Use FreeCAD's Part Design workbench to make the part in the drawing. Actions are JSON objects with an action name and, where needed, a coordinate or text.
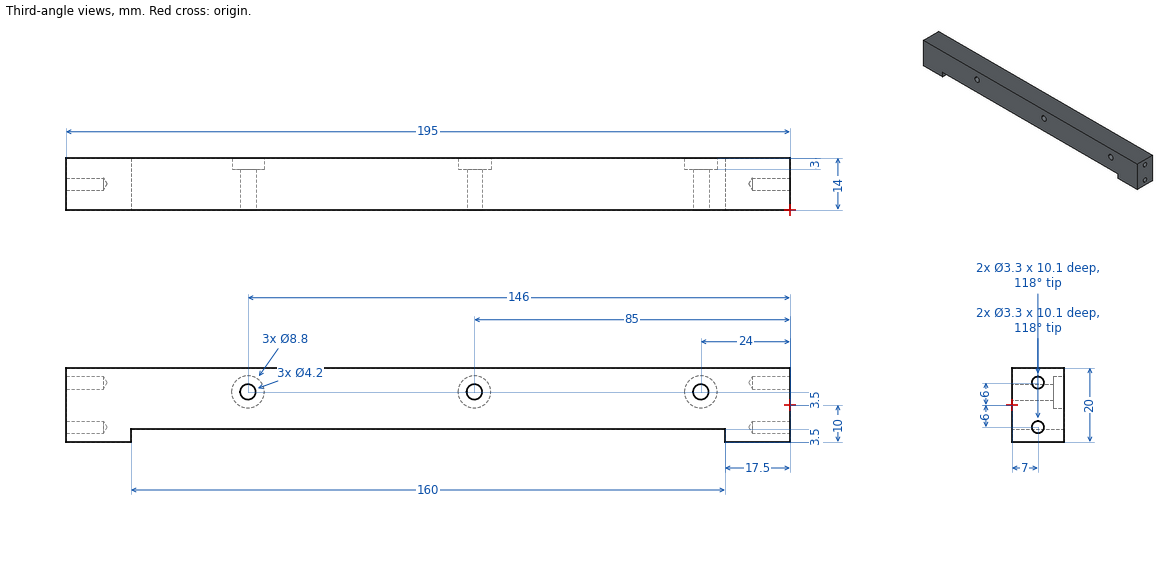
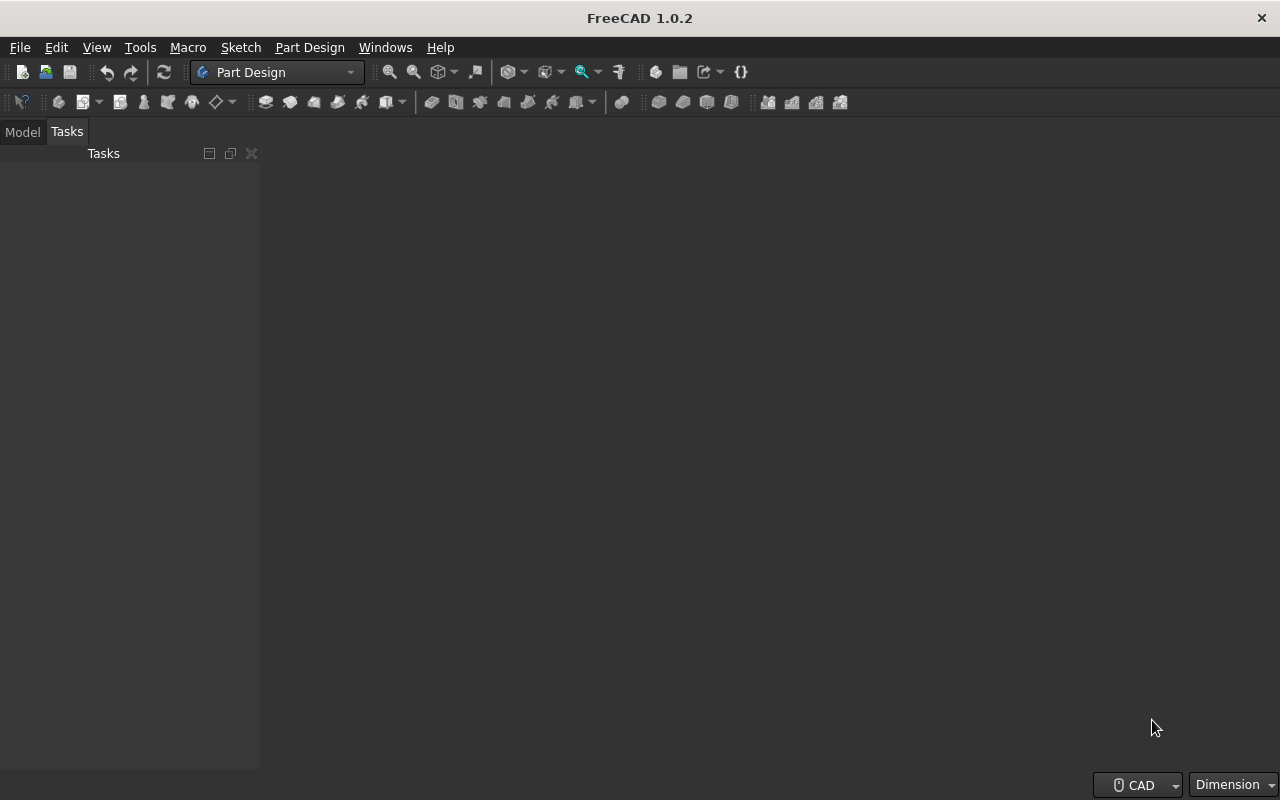
{"action": "left_click", "coordinate": [22, 72]}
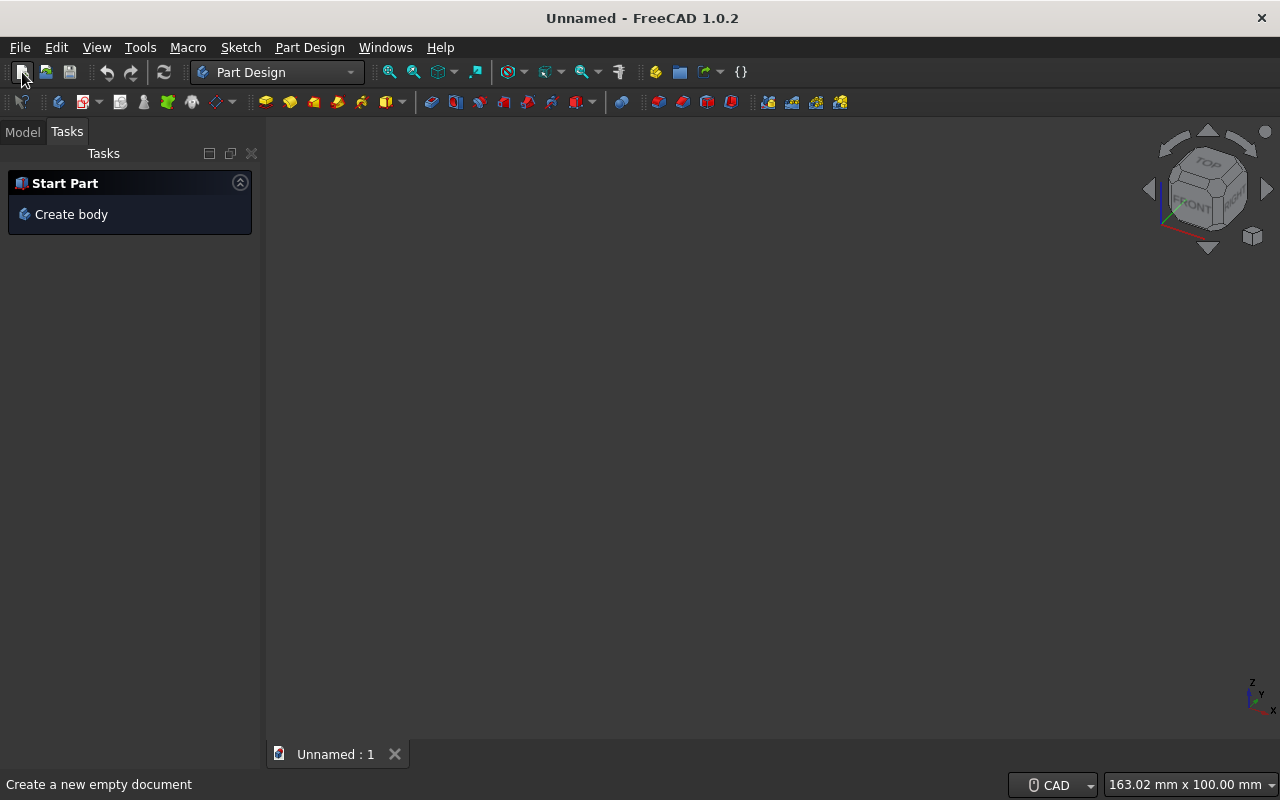
{"action": "left_click", "coordinate": [84, 102]}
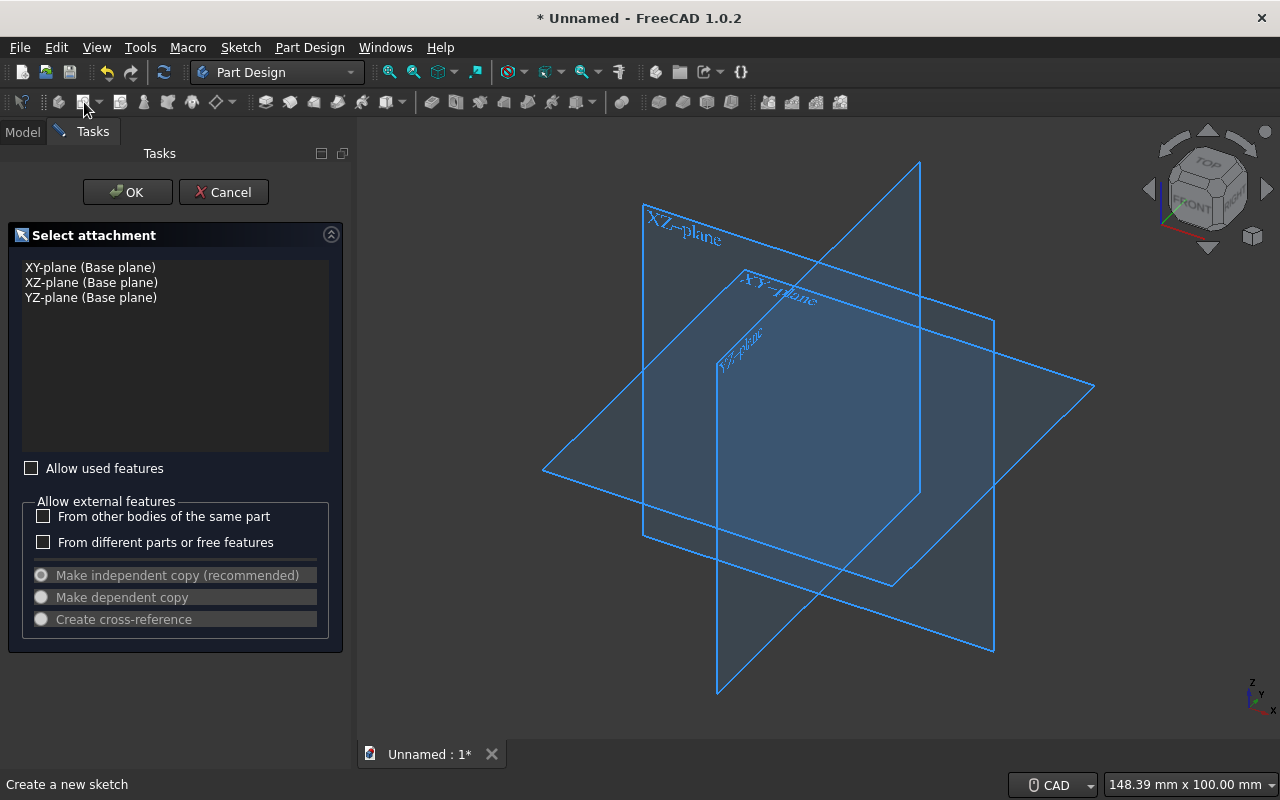
{"action": "left_click", "coordinate": [82, 268]}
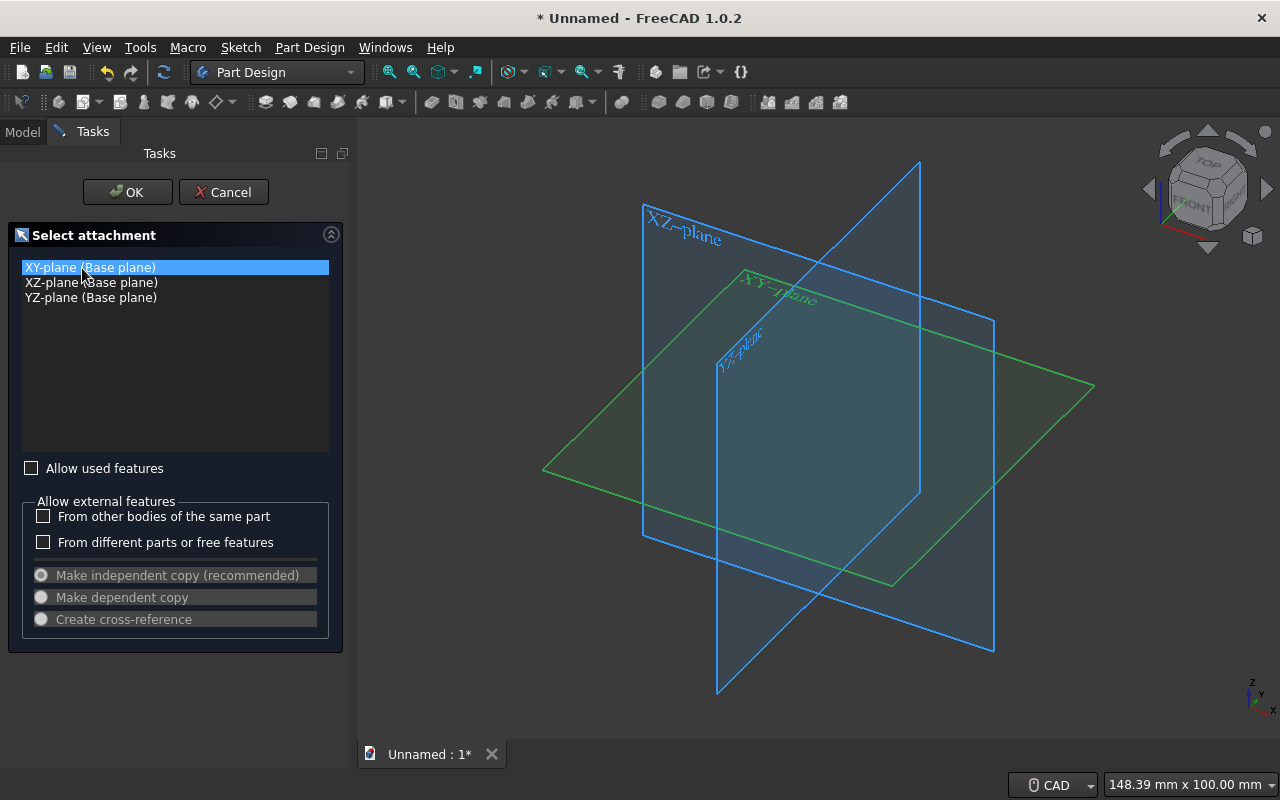
{"action": "left_click", "coordinate": [128, 192]}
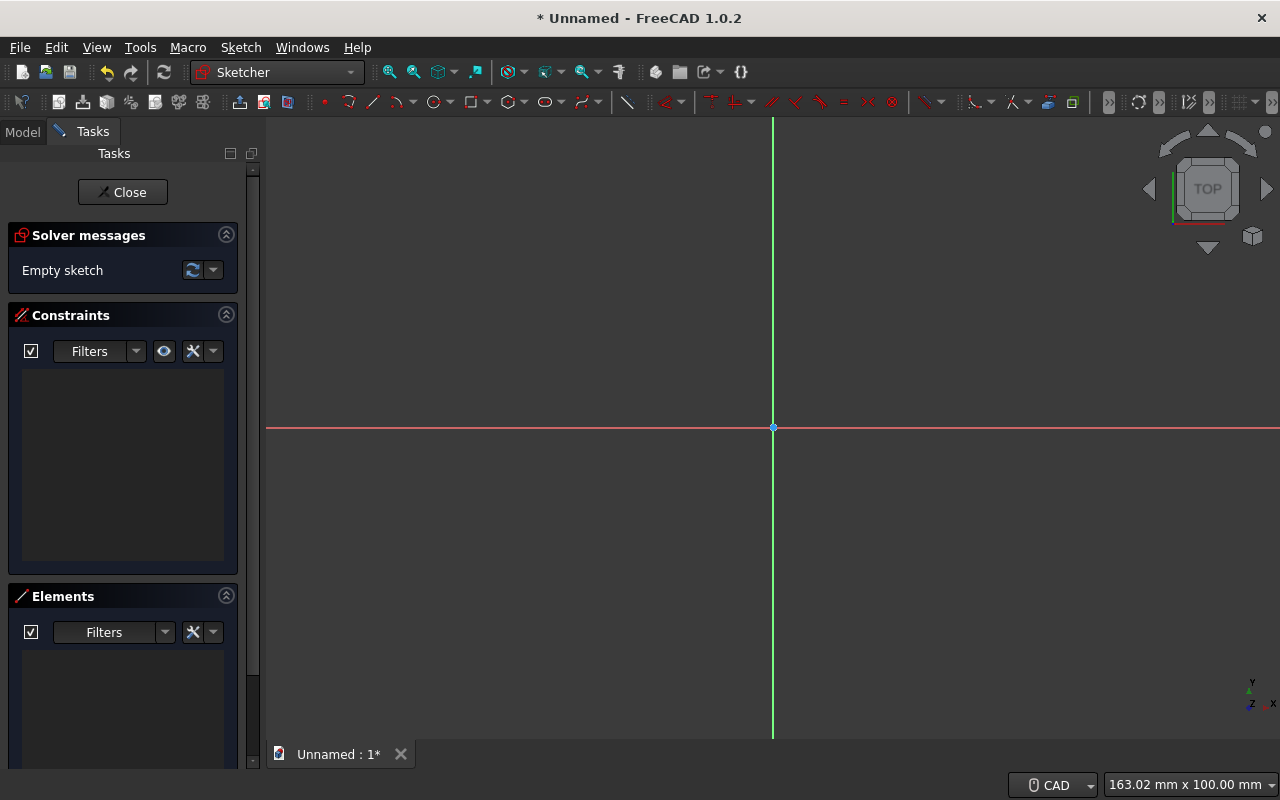
{"action": "scroll", "coordinate": [1115, 464], "scroll_direction": "down", "scroll_amount": 4}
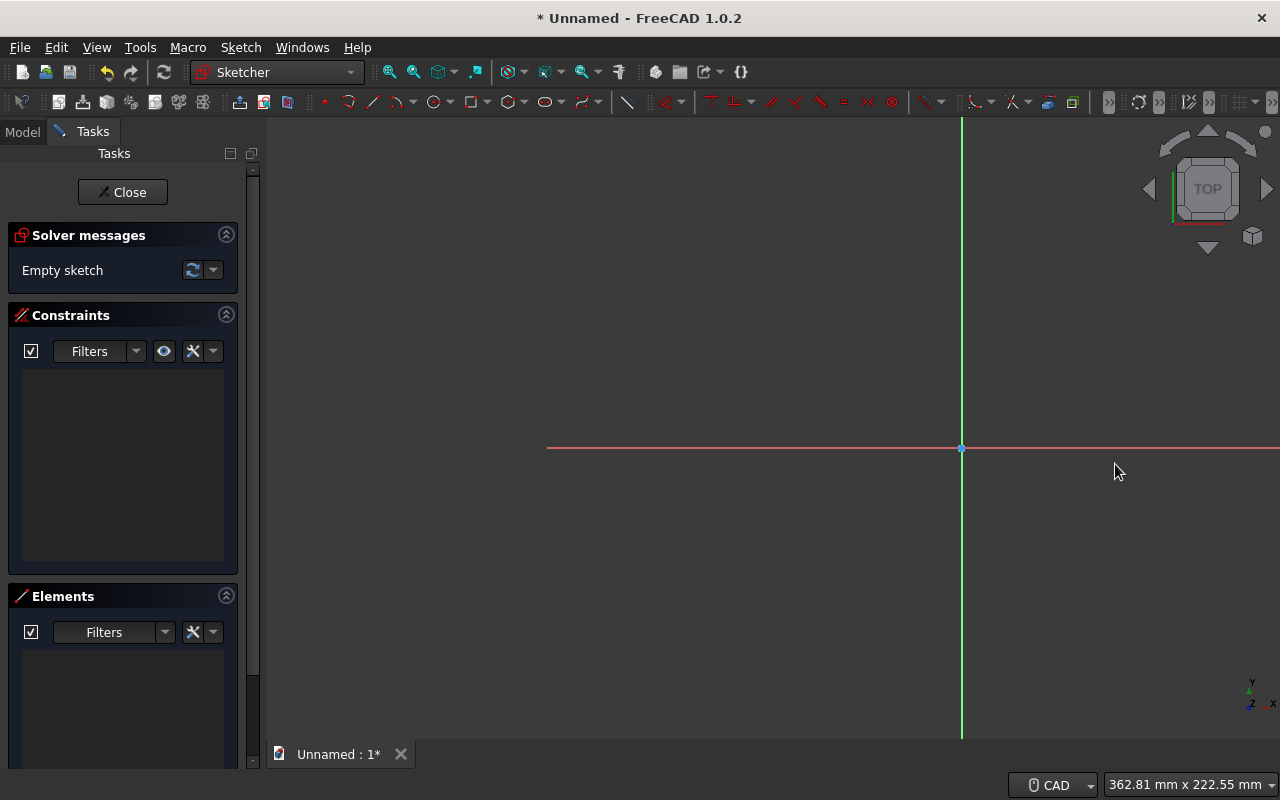
{"action": "key", "text": "g r"}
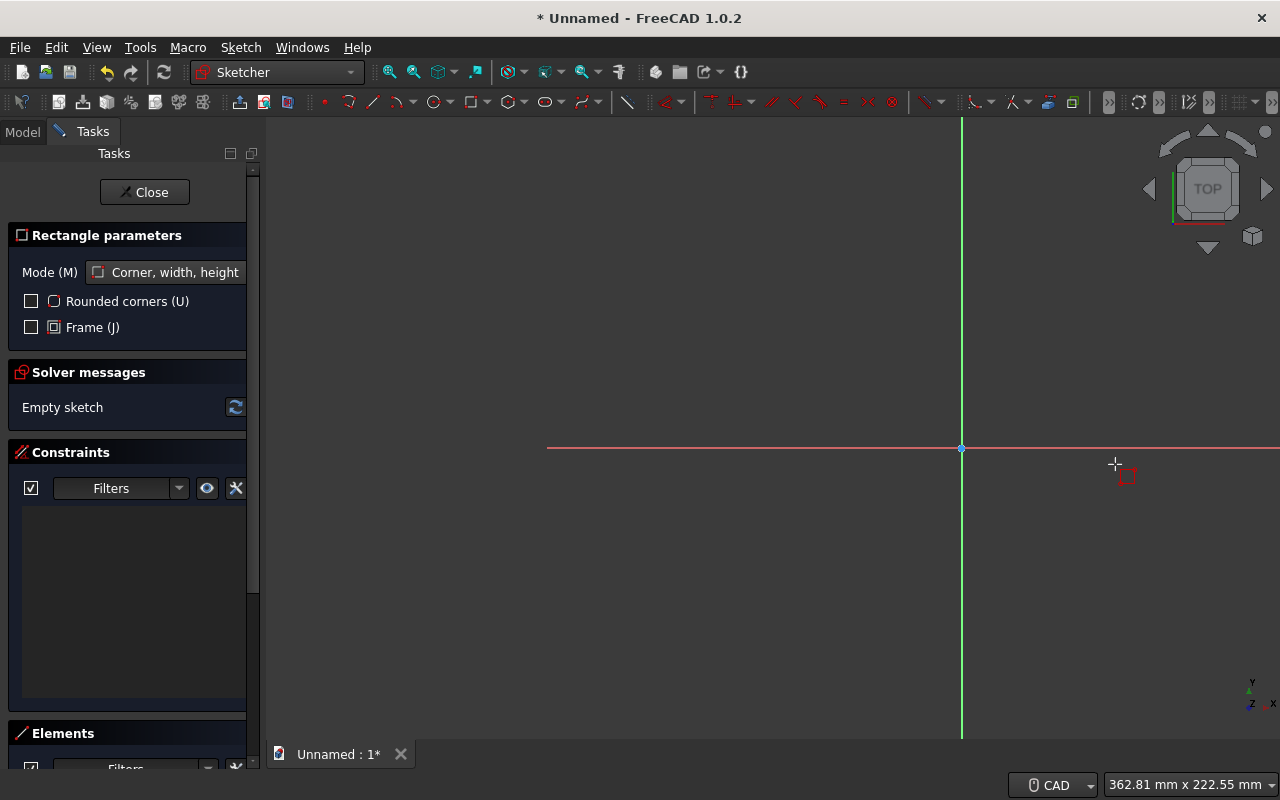
{"action": "left_click", "coordinate": [962, 448]}
{"action": "left_click", "coordinate": [417, 409]}
{"action": "key", "text": "Escape"}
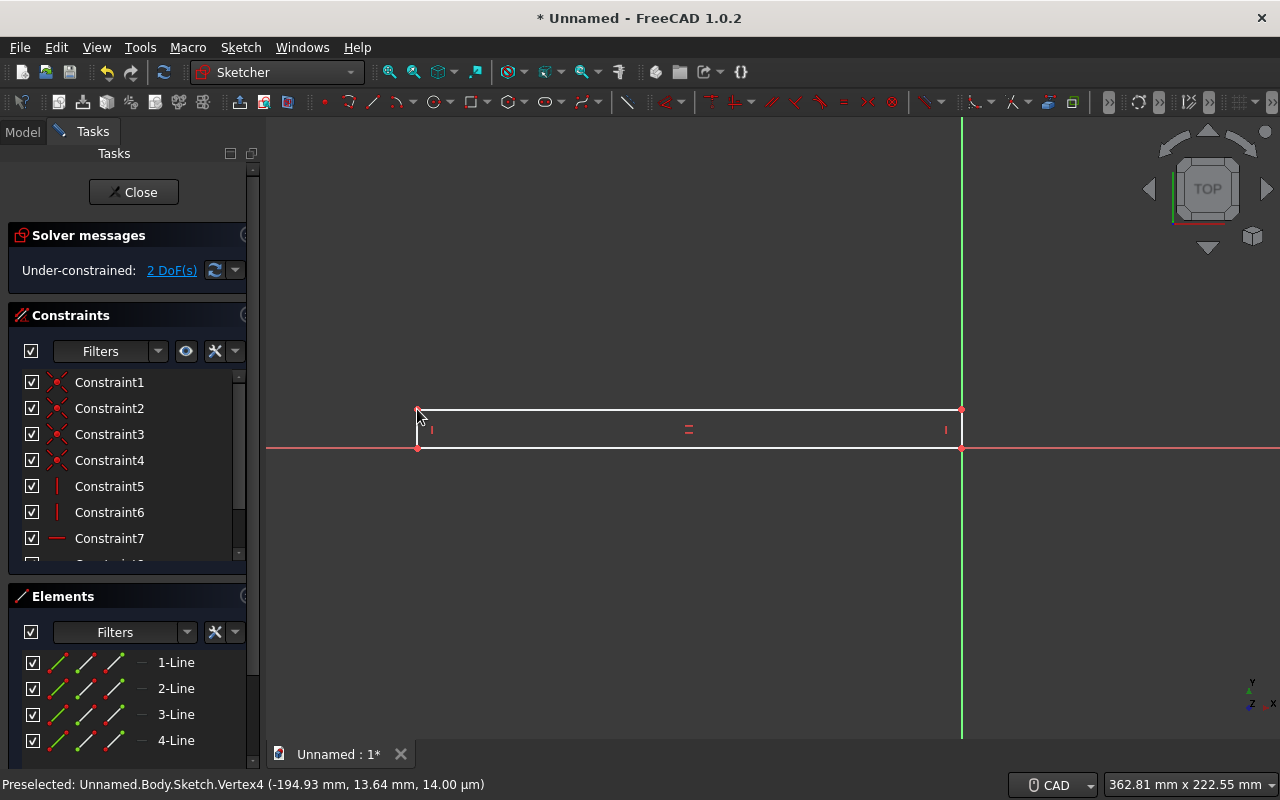
{"action": "left_click", "coordinate": [962, 437]}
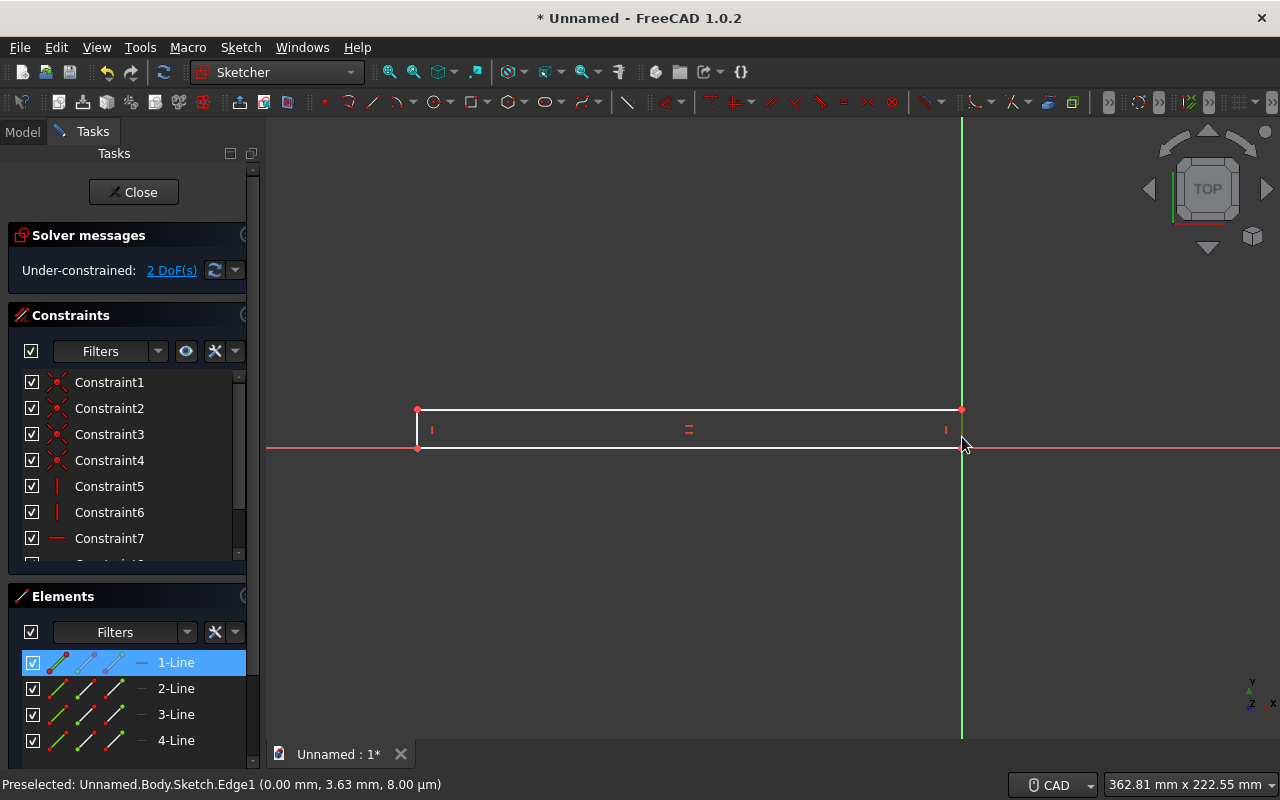
{"action": "key", "text": "i"}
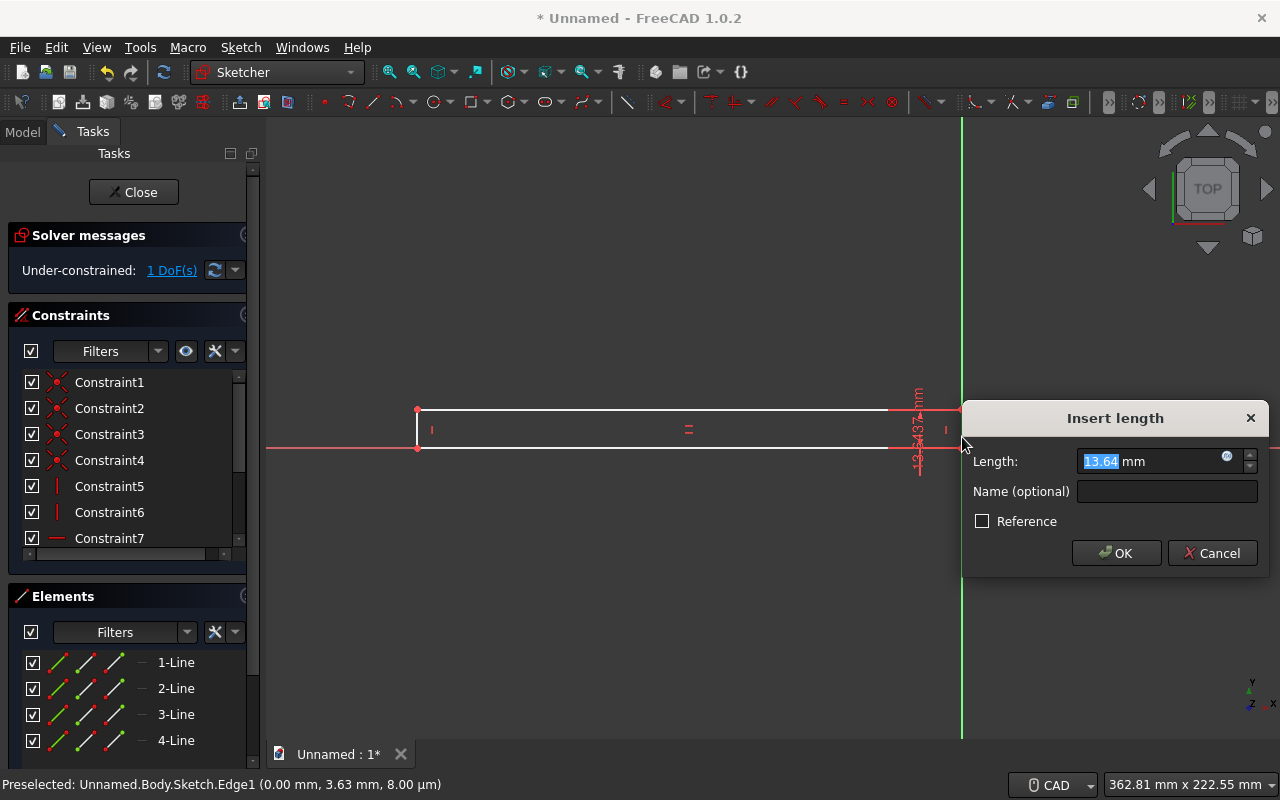
{"action": "type", "text": "14"}
{"action": "key", "text": "Return"}